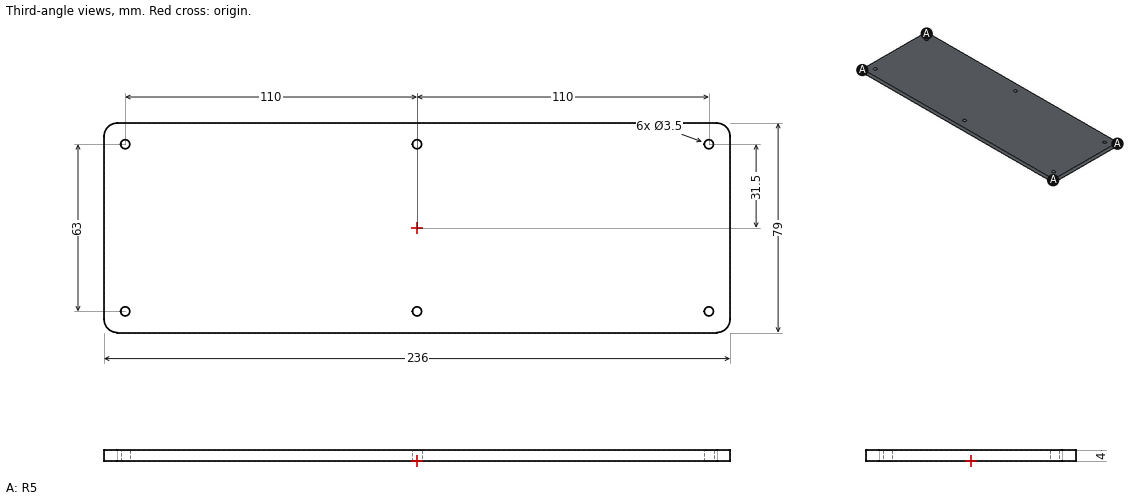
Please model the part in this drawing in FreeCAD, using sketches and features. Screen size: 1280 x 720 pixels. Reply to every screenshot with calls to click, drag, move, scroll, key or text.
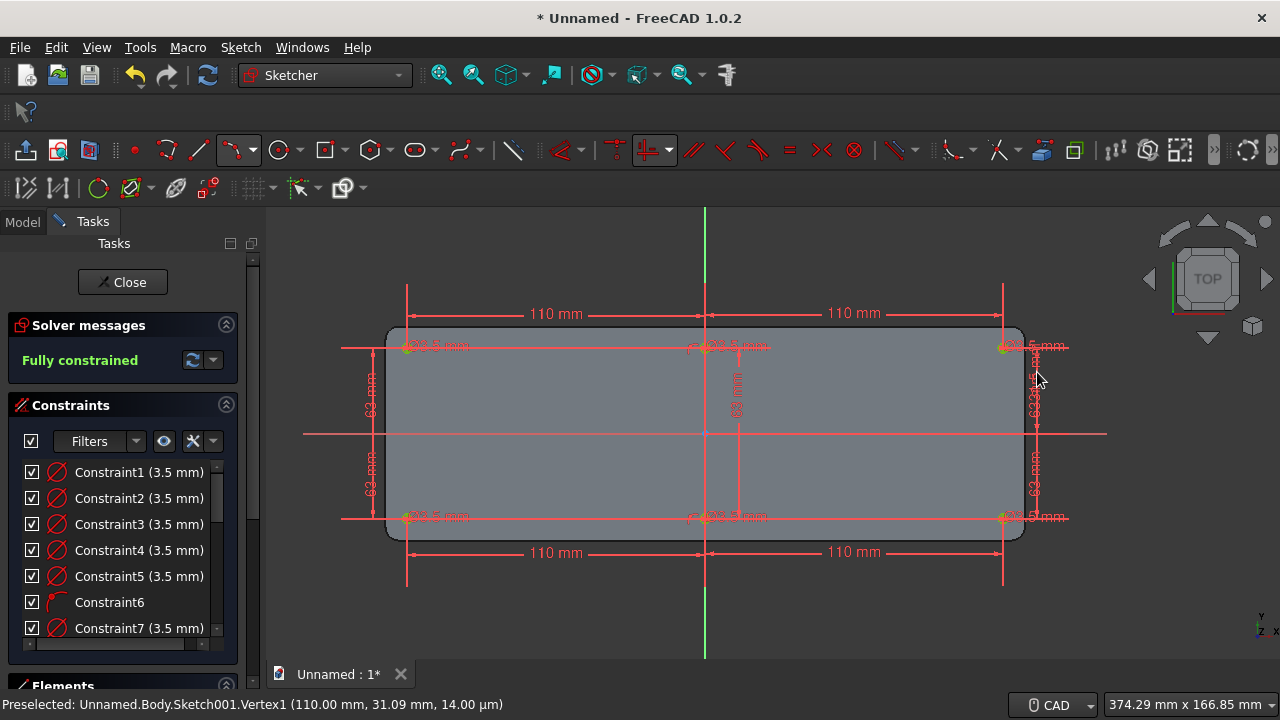
click(123, 282)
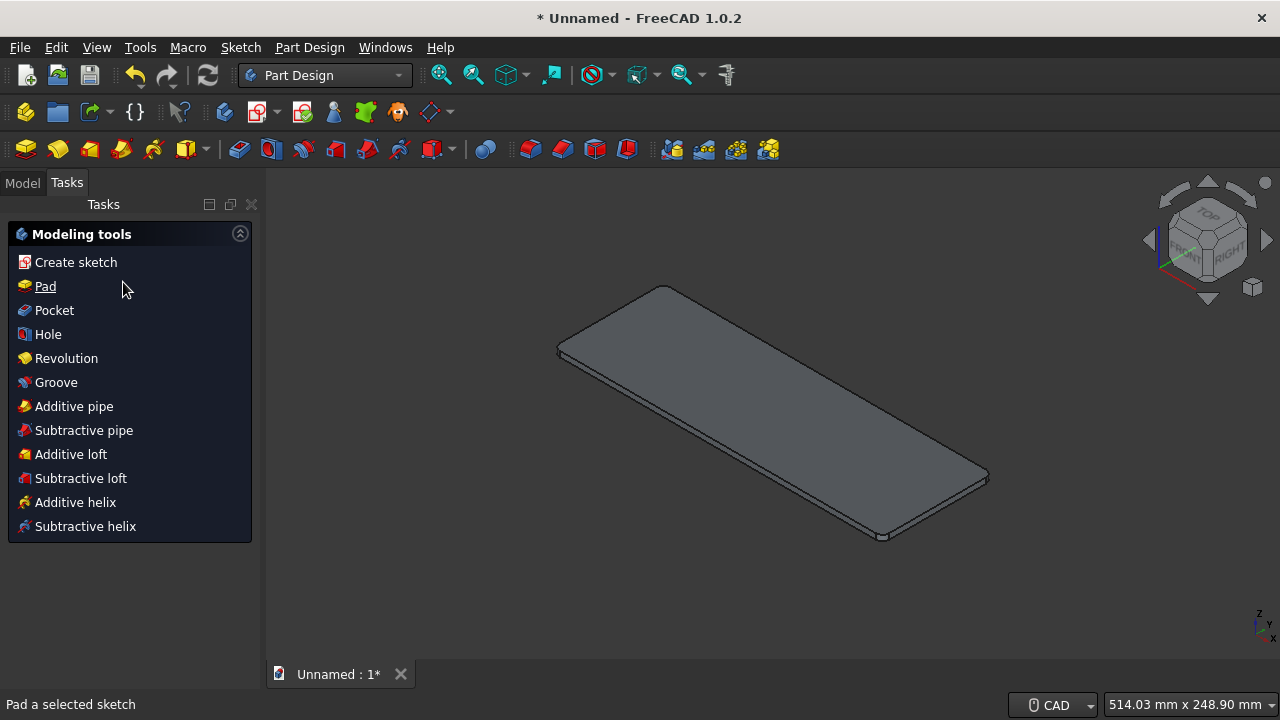
click(240, 150)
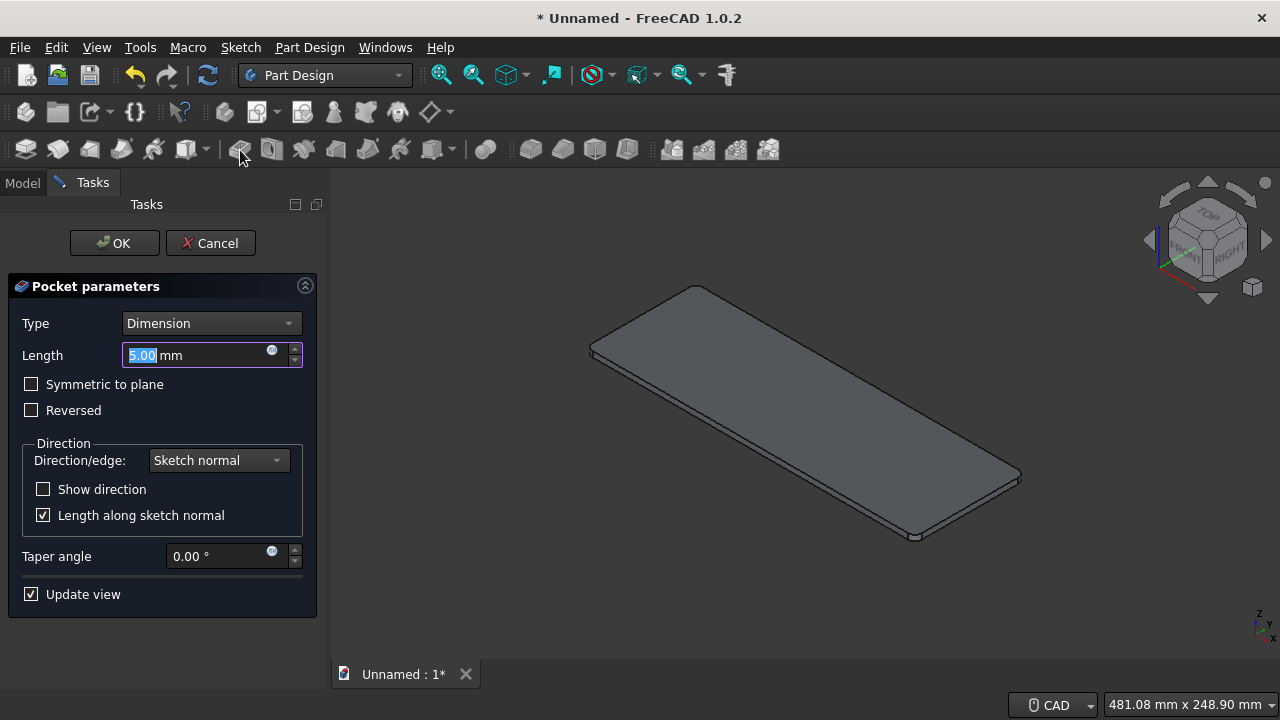
click(212, 324)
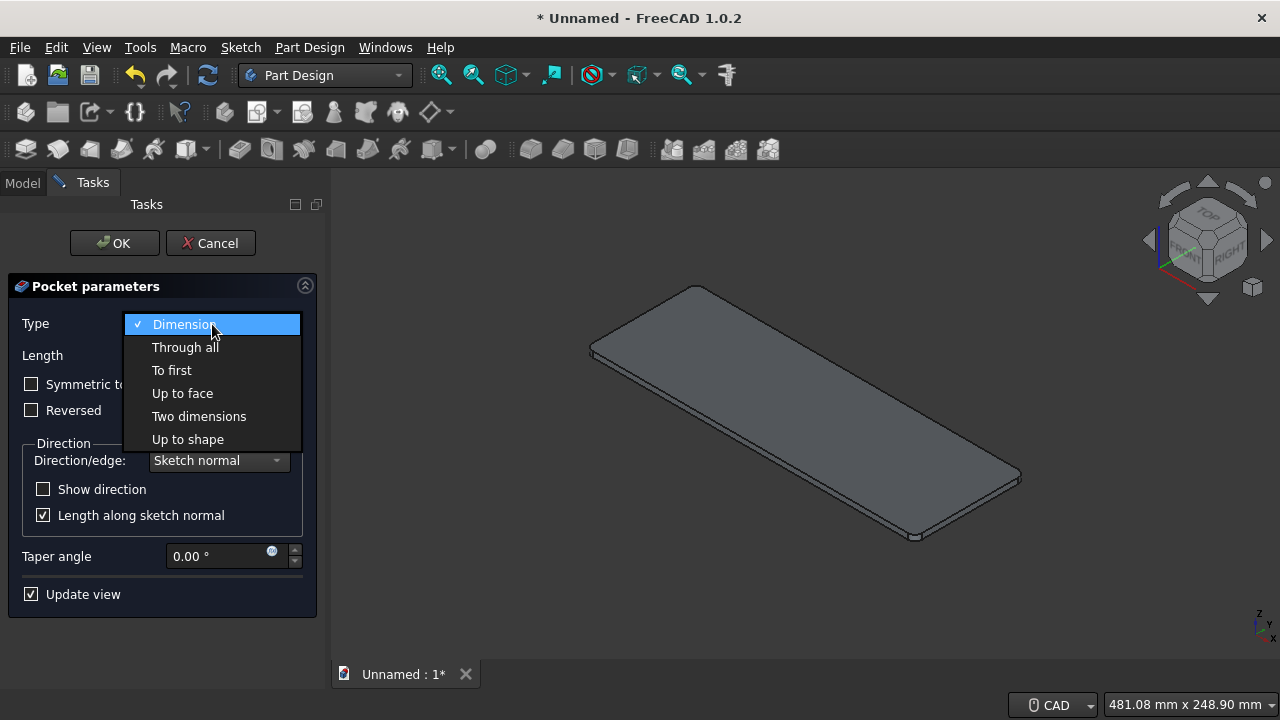
click(212, 348)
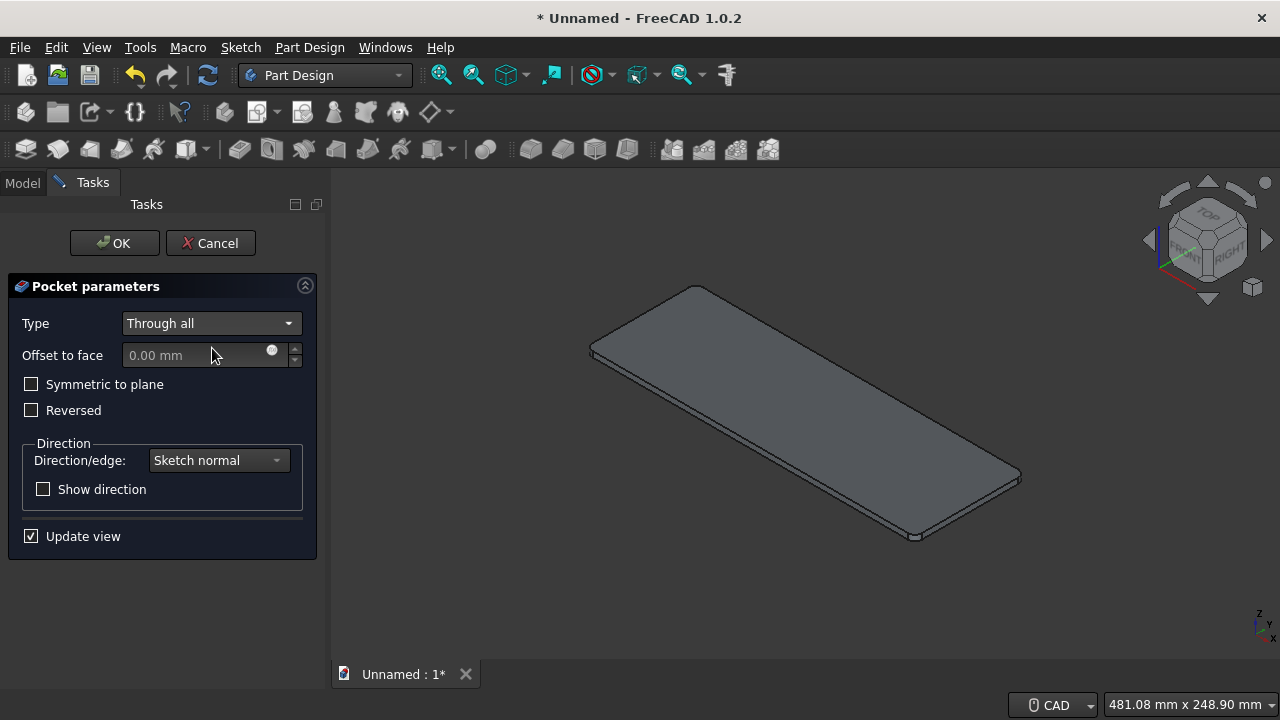
click(30, 410)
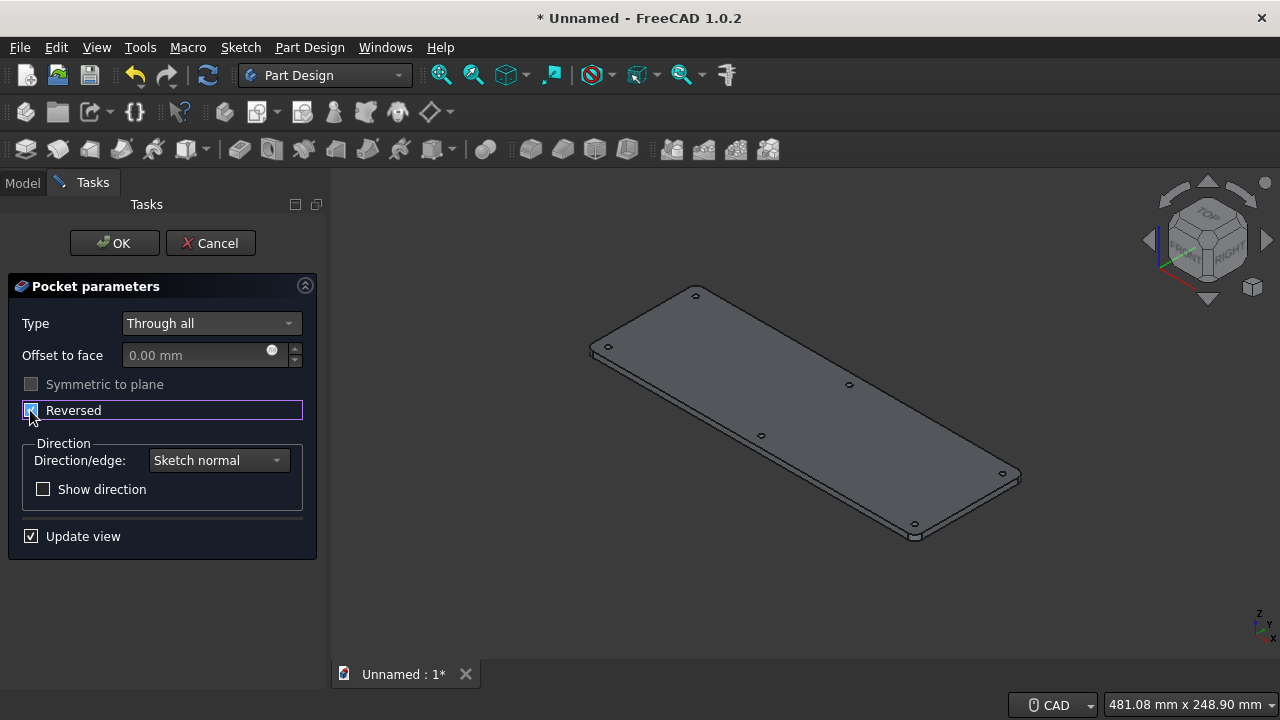
click(115, 243)